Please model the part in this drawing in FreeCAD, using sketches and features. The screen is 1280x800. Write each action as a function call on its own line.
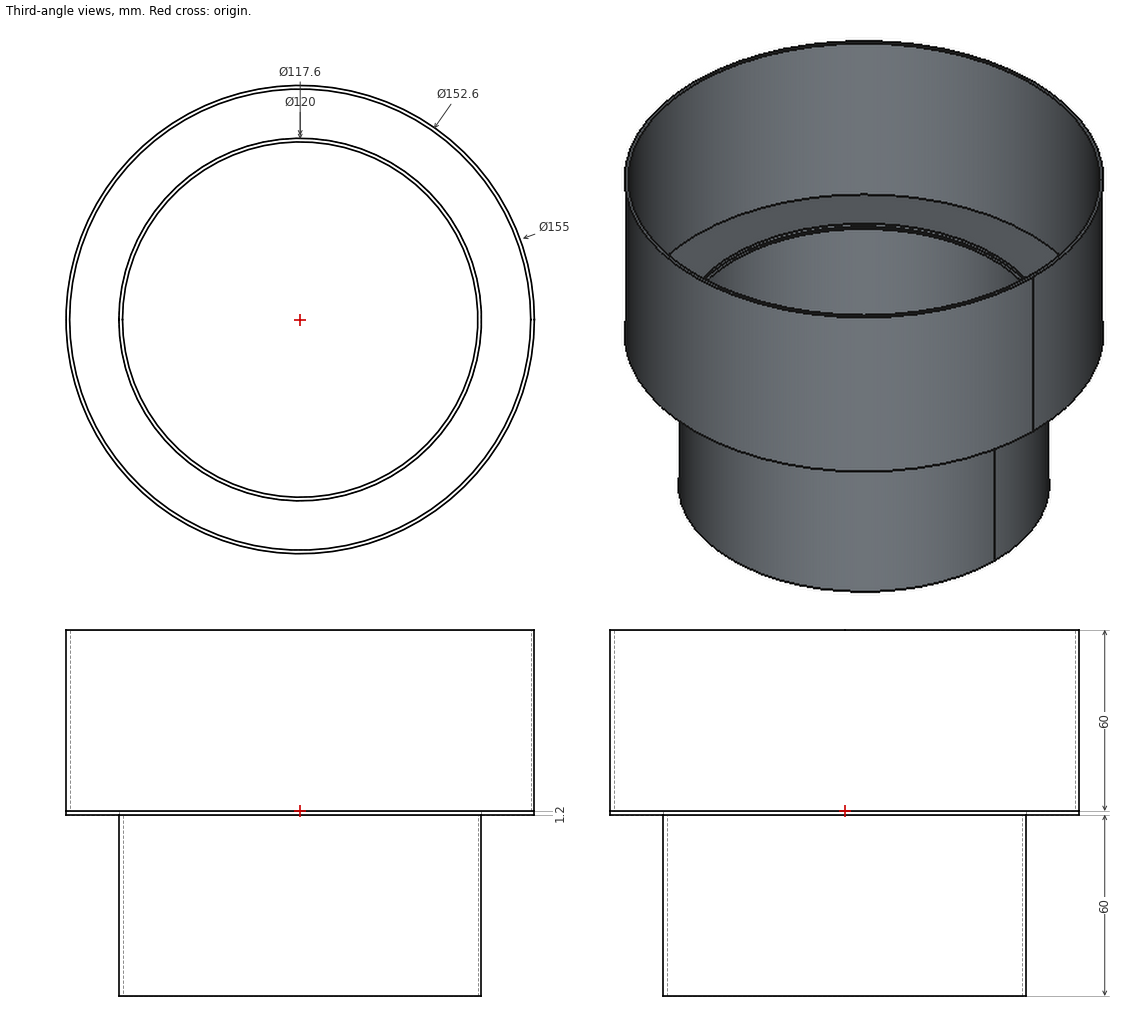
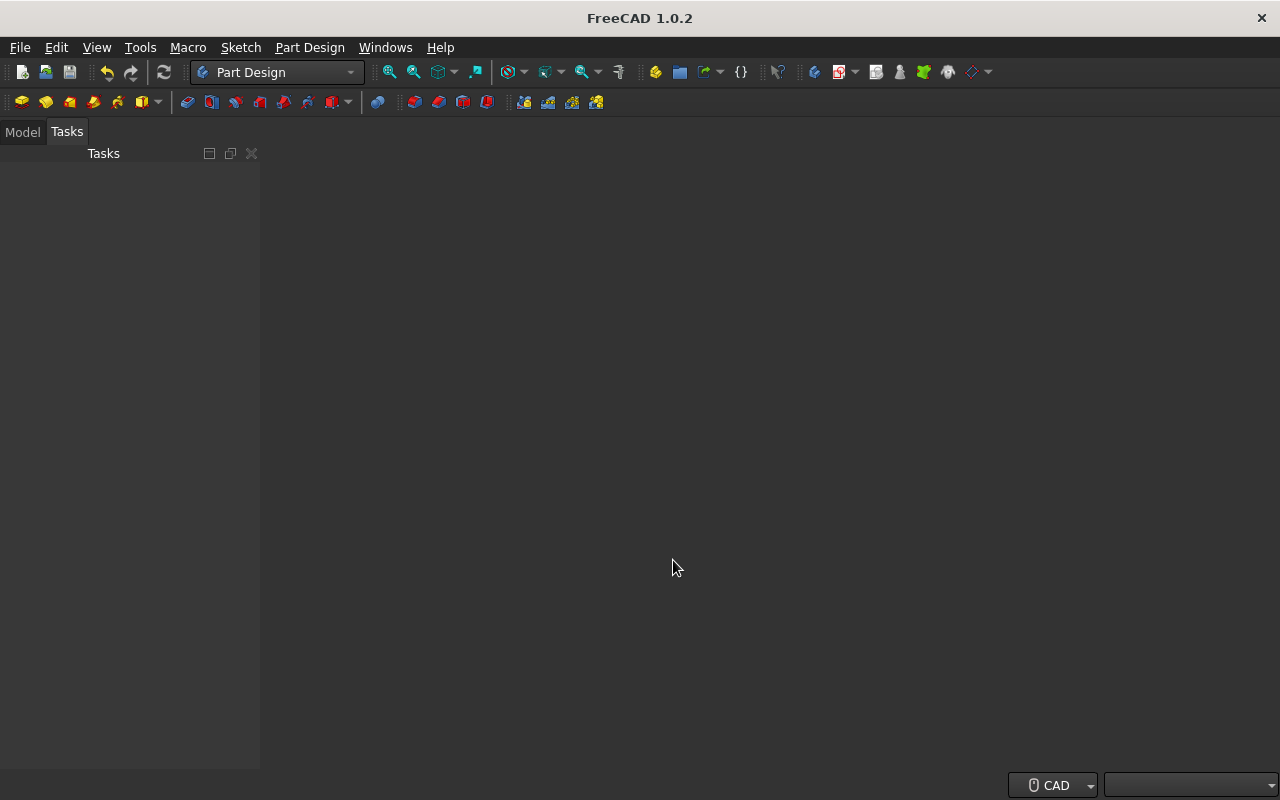
click(22, 72)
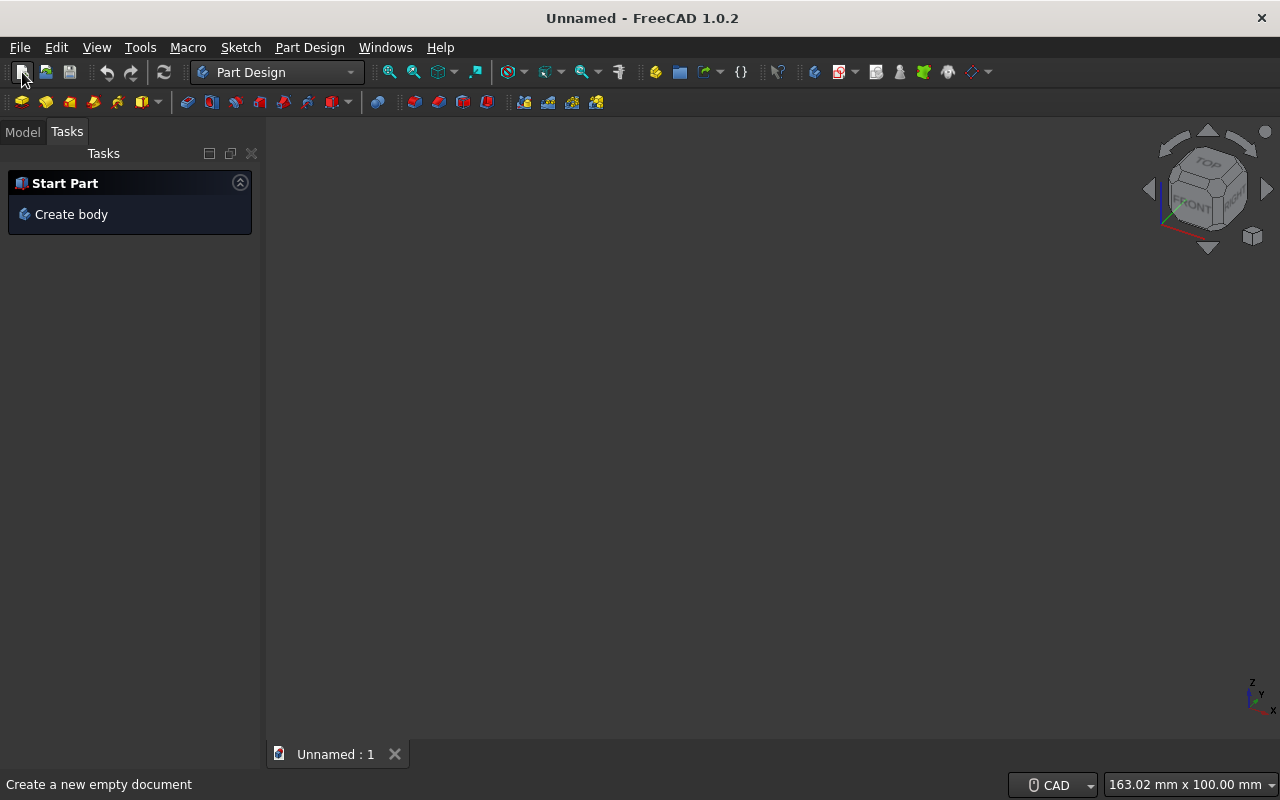
click(840, 72)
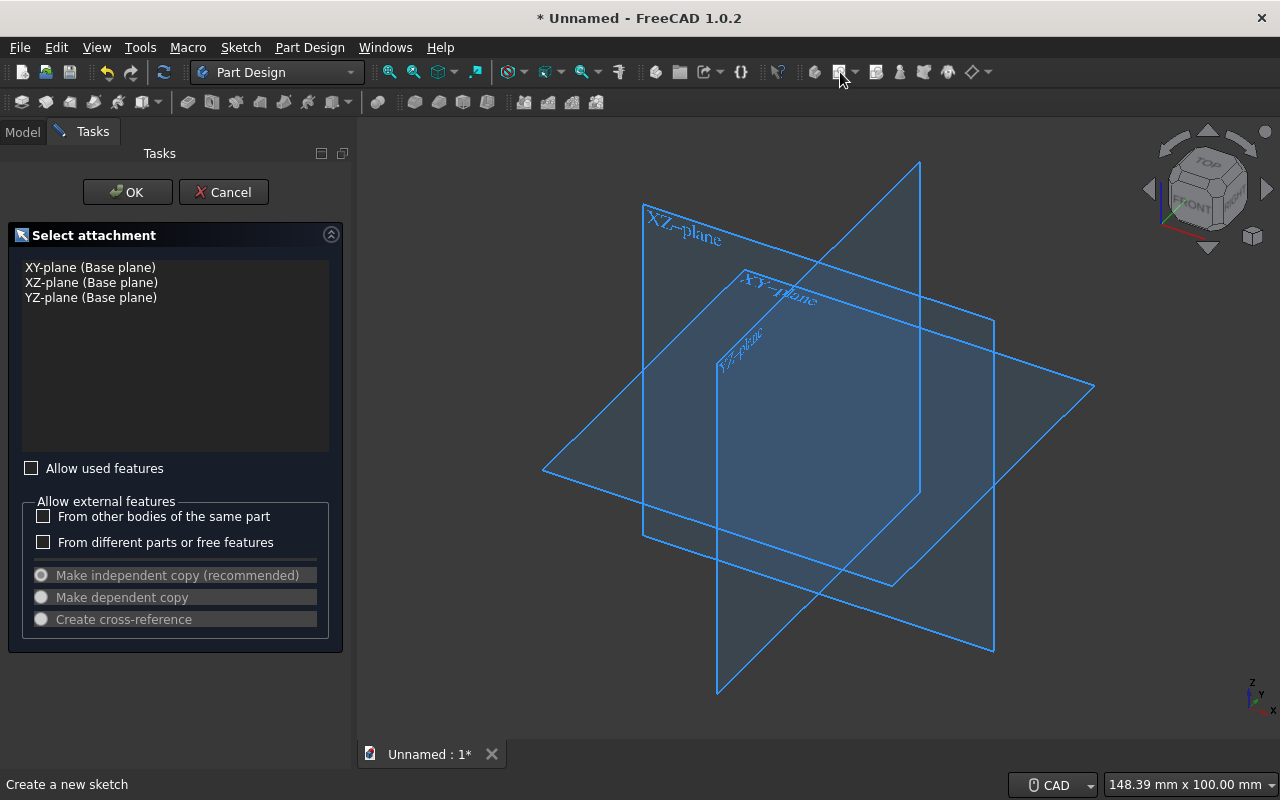
click(82, 268)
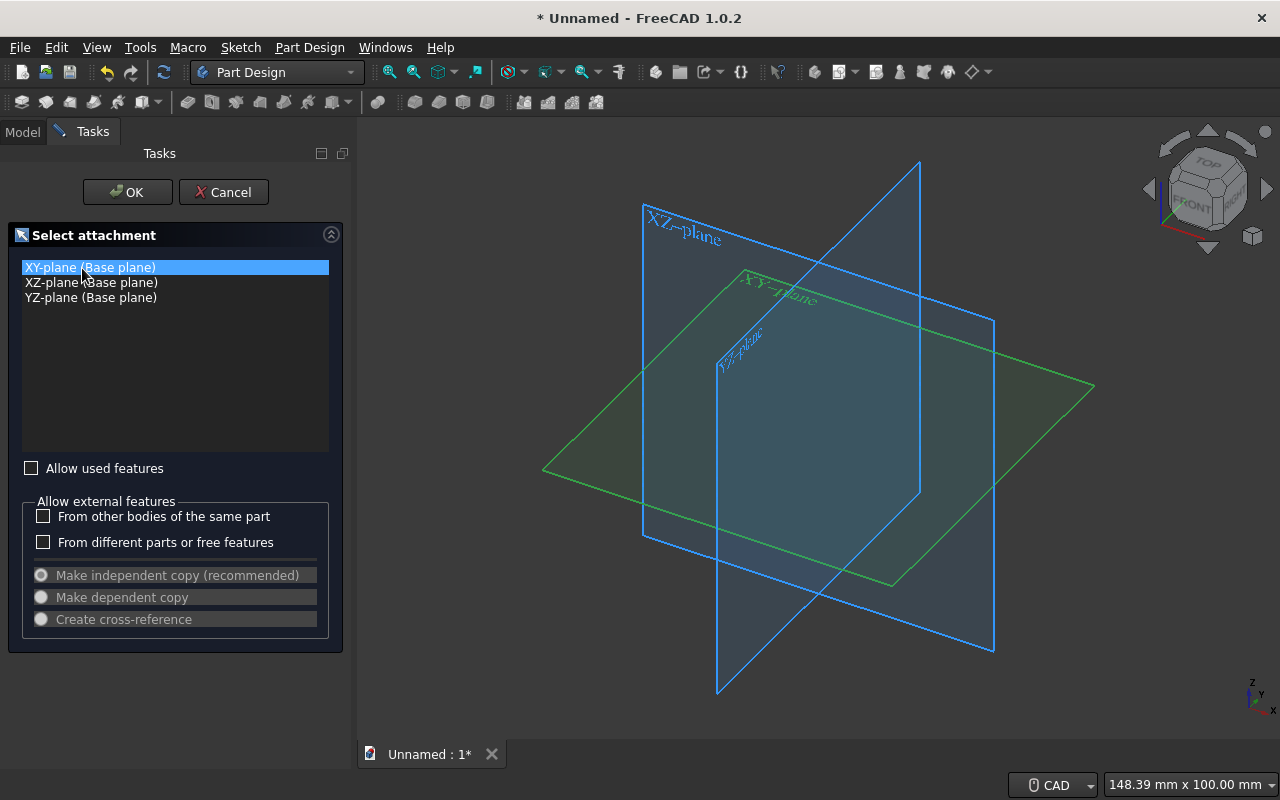
click(128, 192)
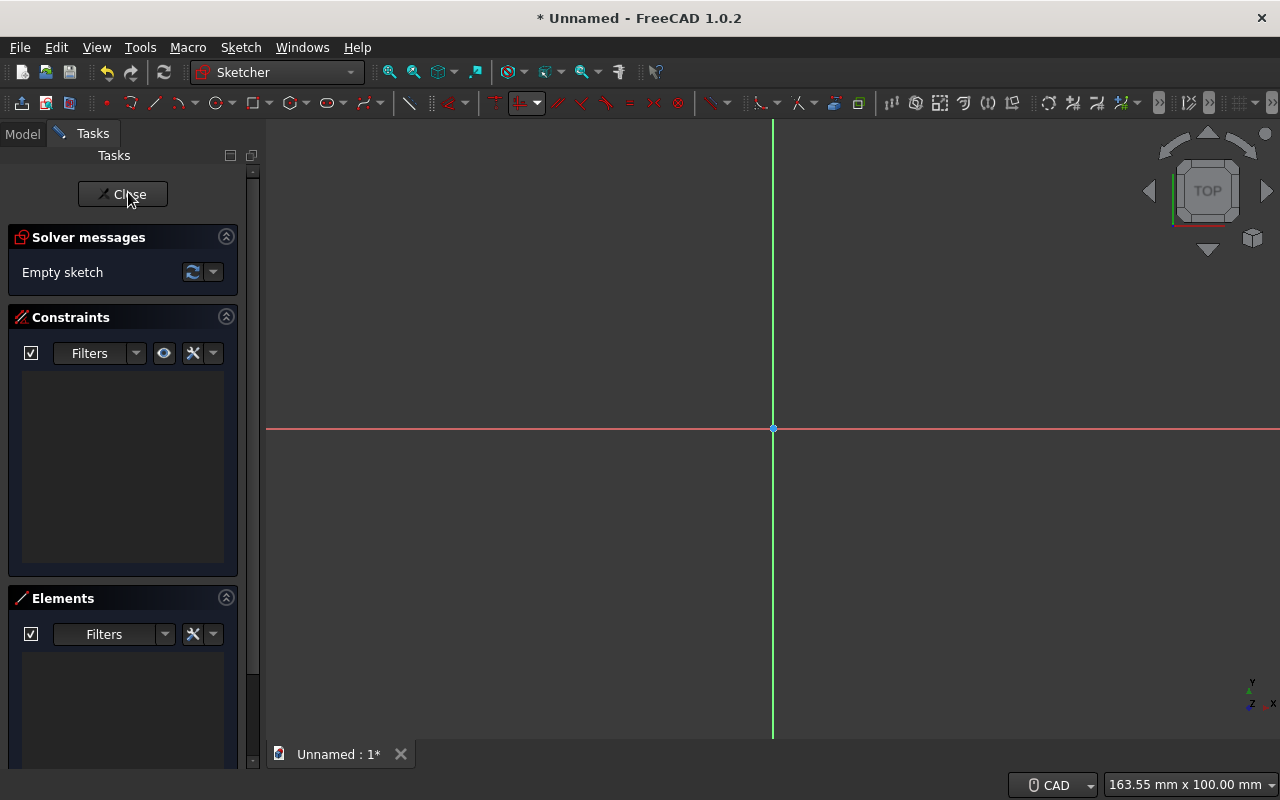
scroll(649, 429, down, 4)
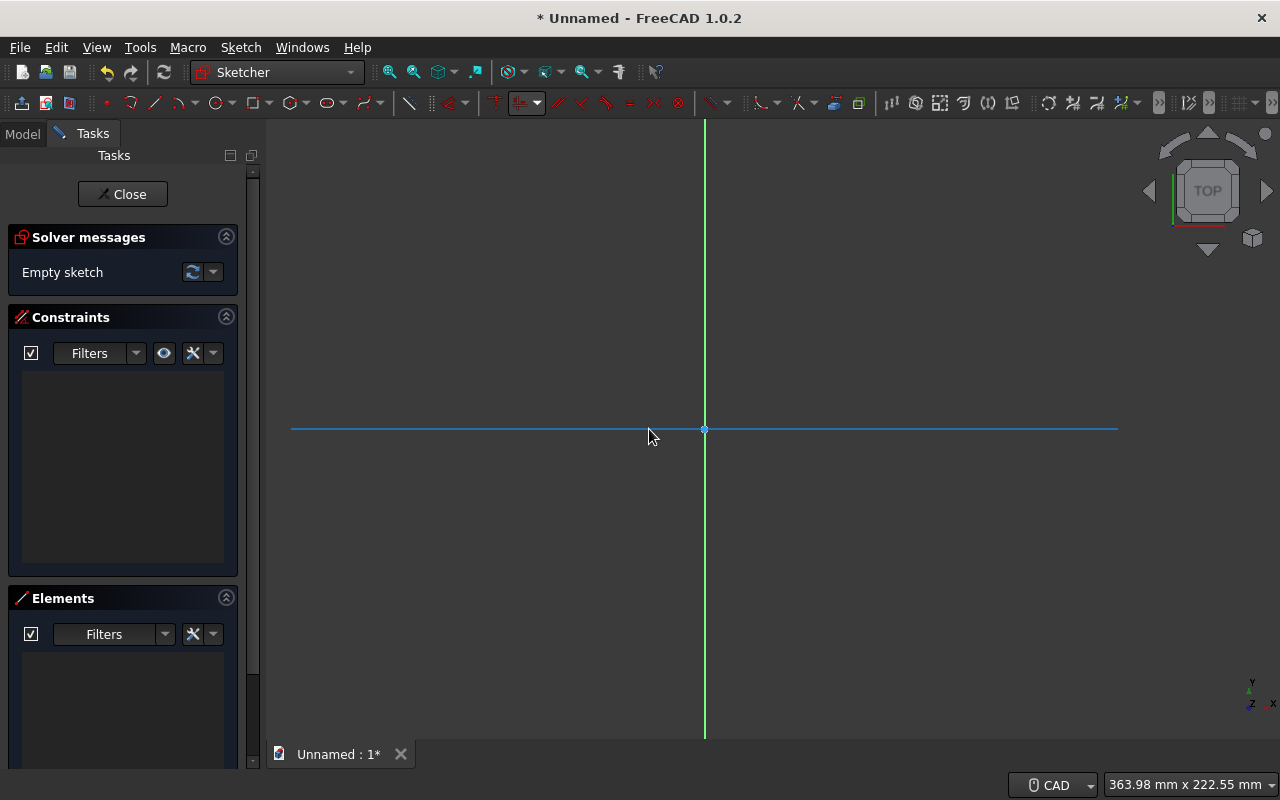
click(216, 104)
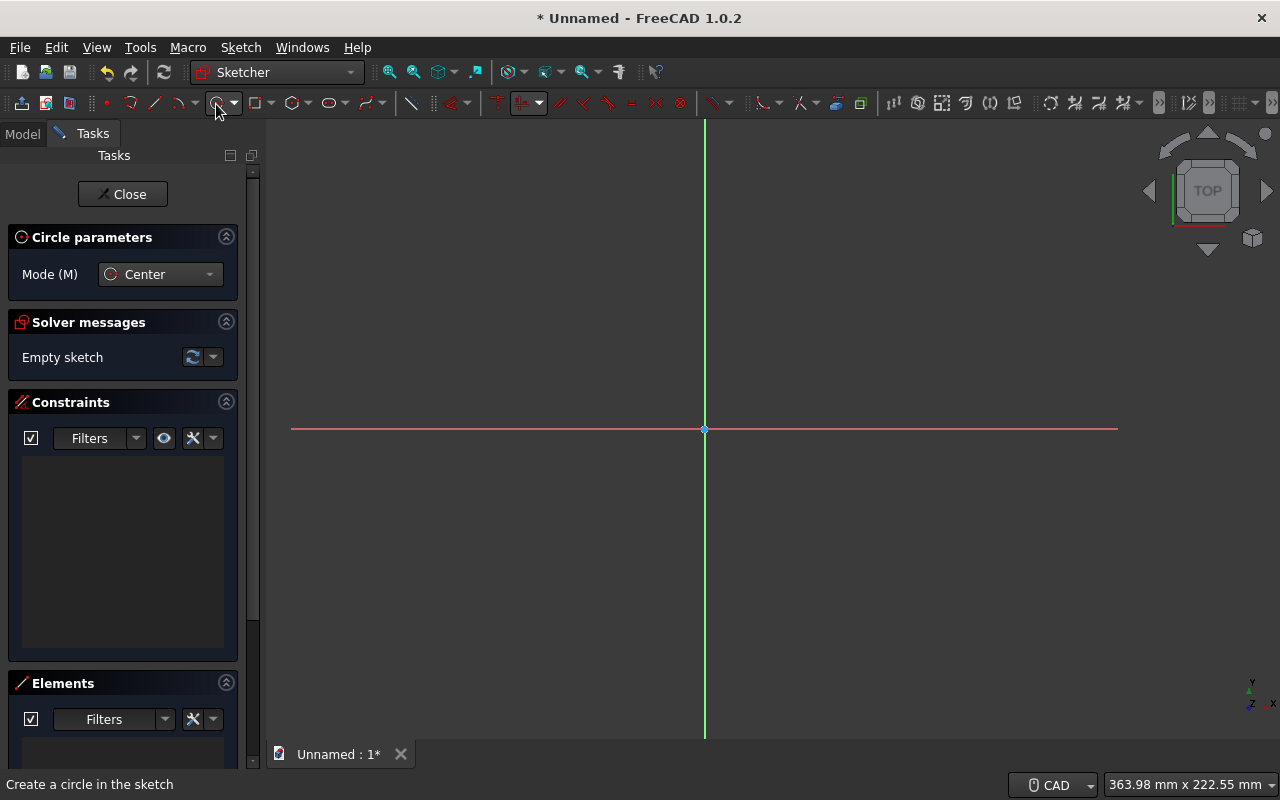
click(705, 429)
click(858, 277)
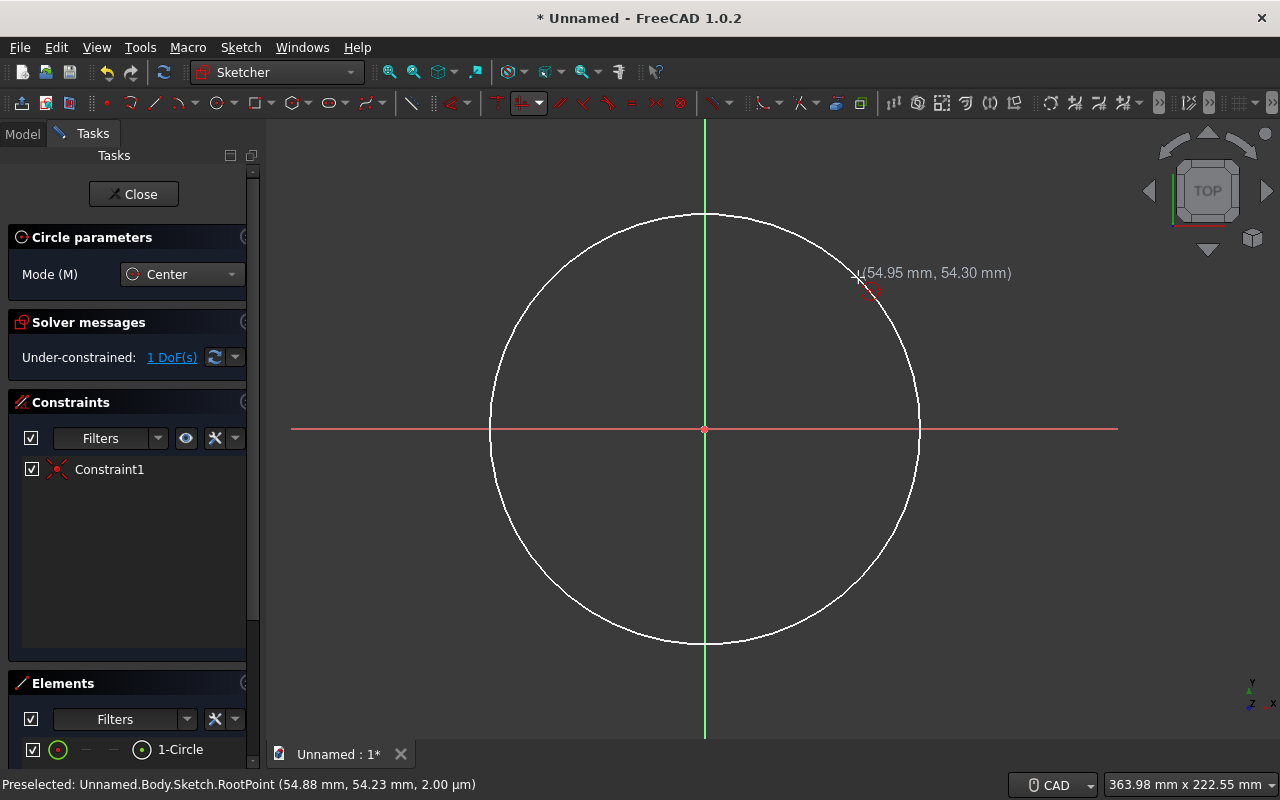
click(705, 429)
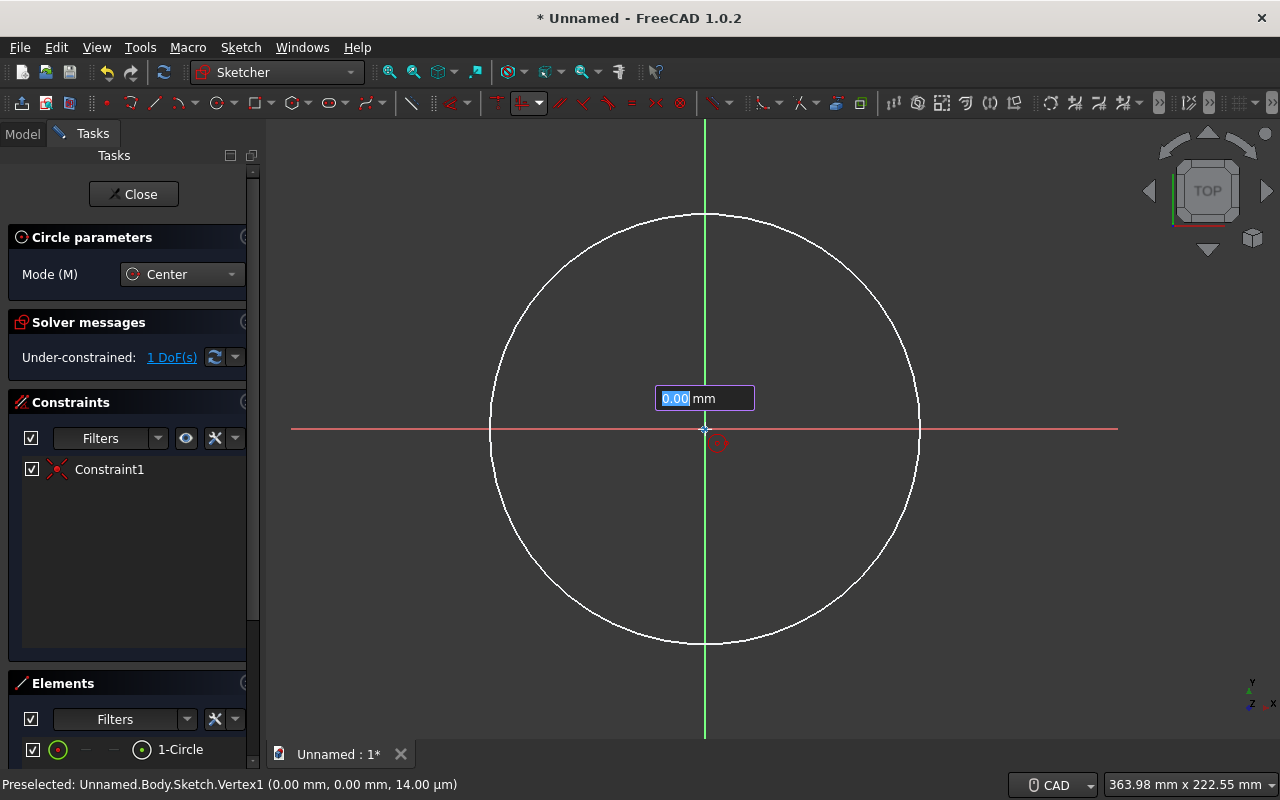
scroll(855, 279, up, 8)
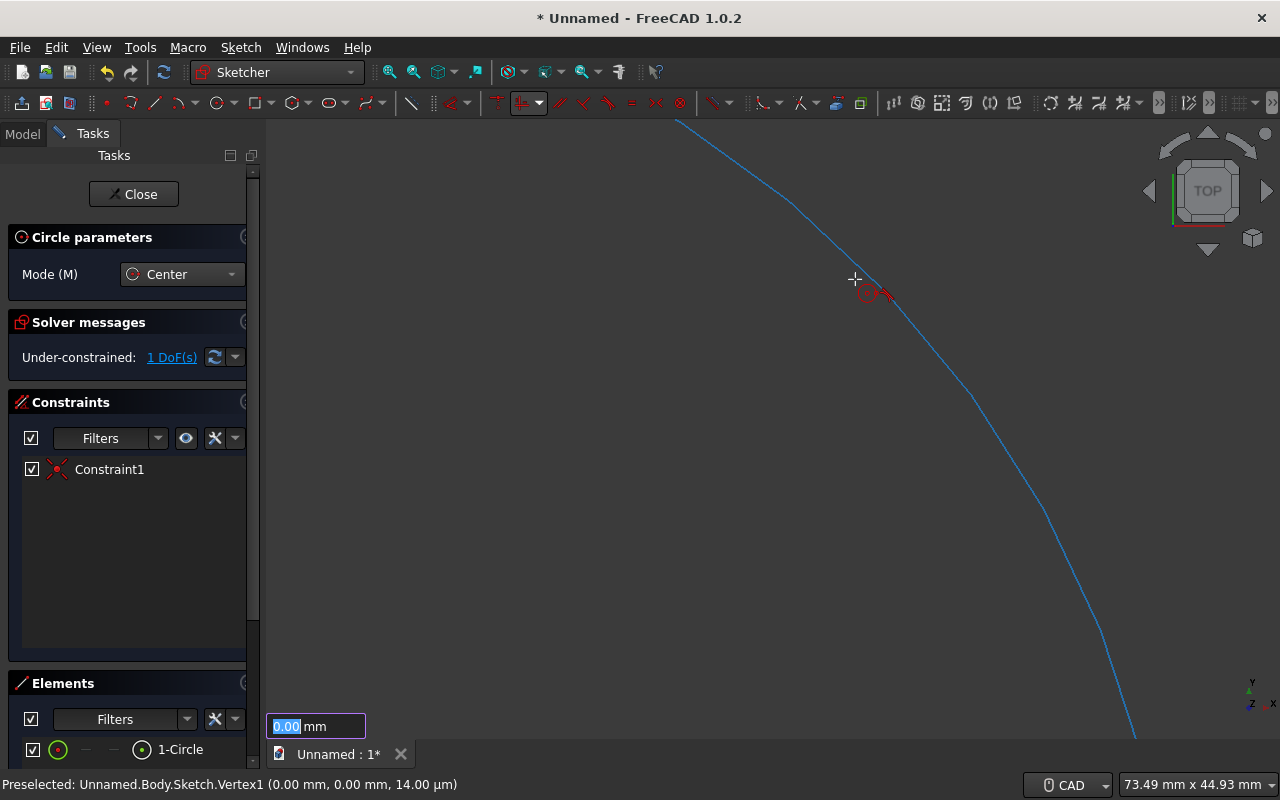
click(854, 278)
key(Escape)